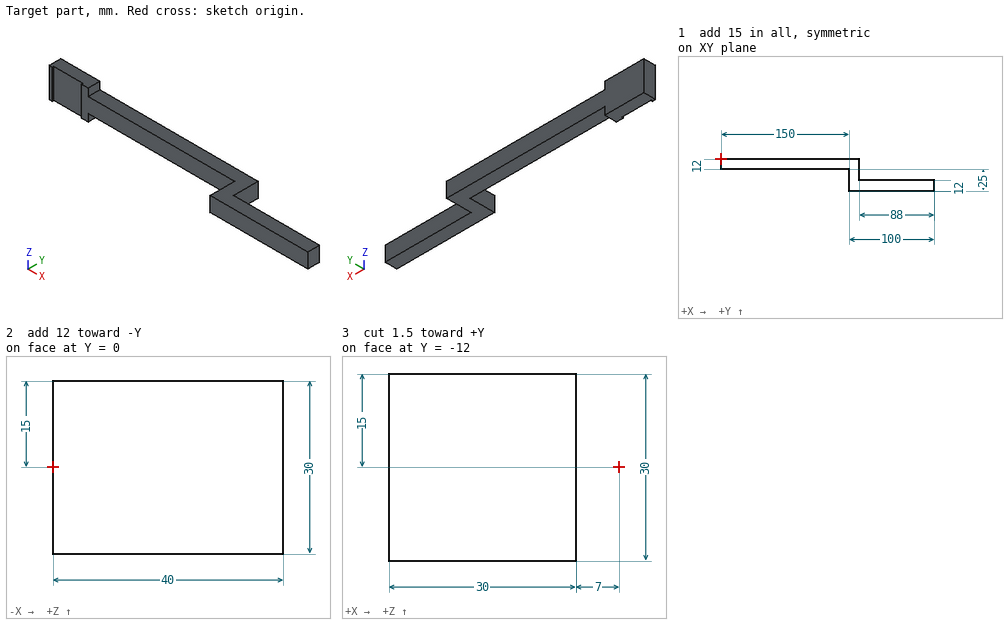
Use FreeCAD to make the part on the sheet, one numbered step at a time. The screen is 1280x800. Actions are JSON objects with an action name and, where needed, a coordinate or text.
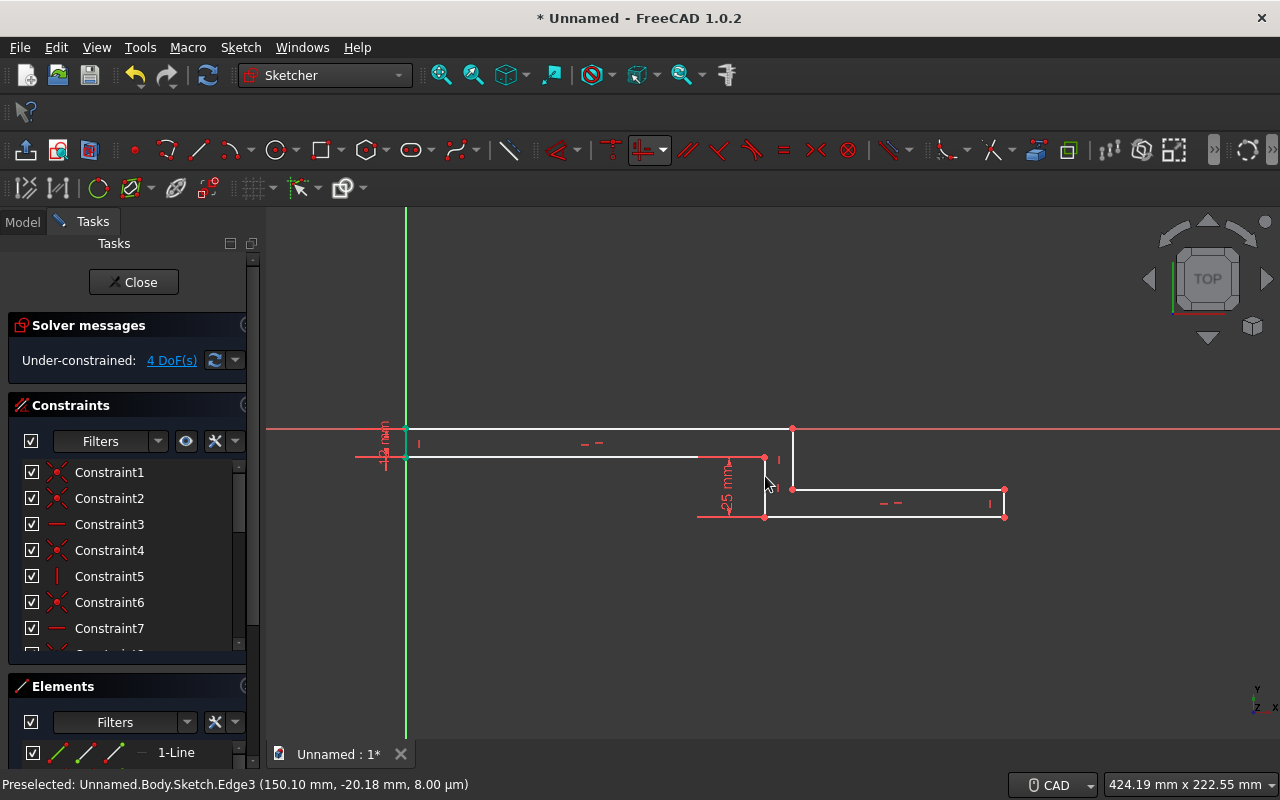
{"action": "scroll", "coordinate": [1004, 506], "scroll_direction": "up", "scroll_amount": 2}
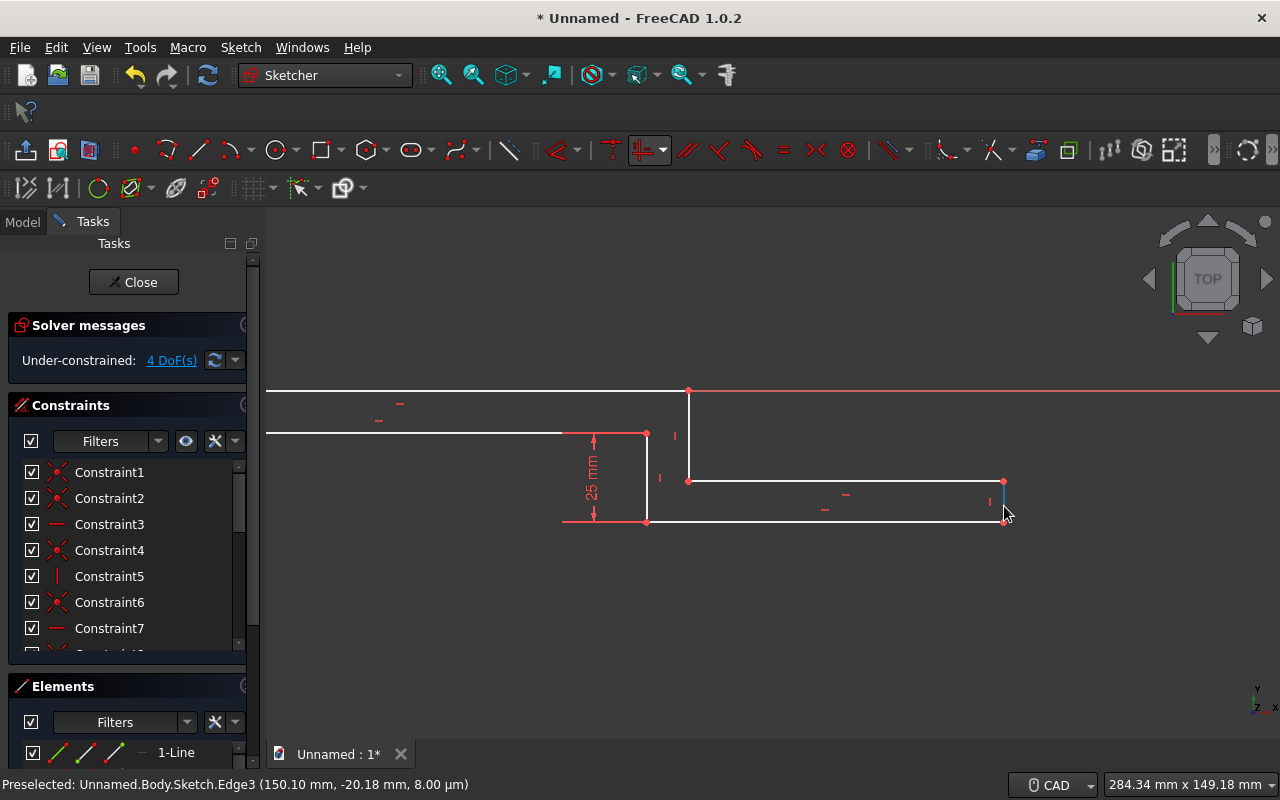
{"action": "left_click", "coordinate": [1004, 506]}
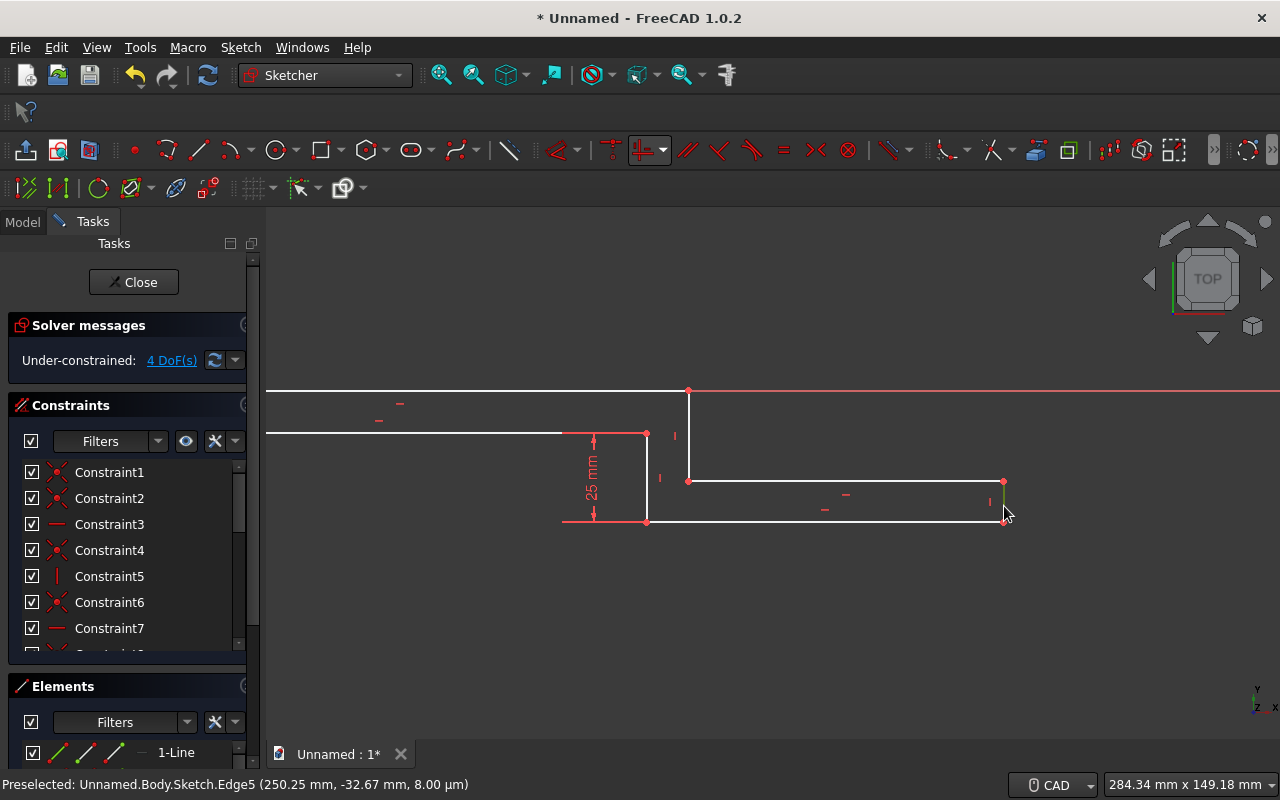
{"action": "left_click", "coordinate": [580, 150]}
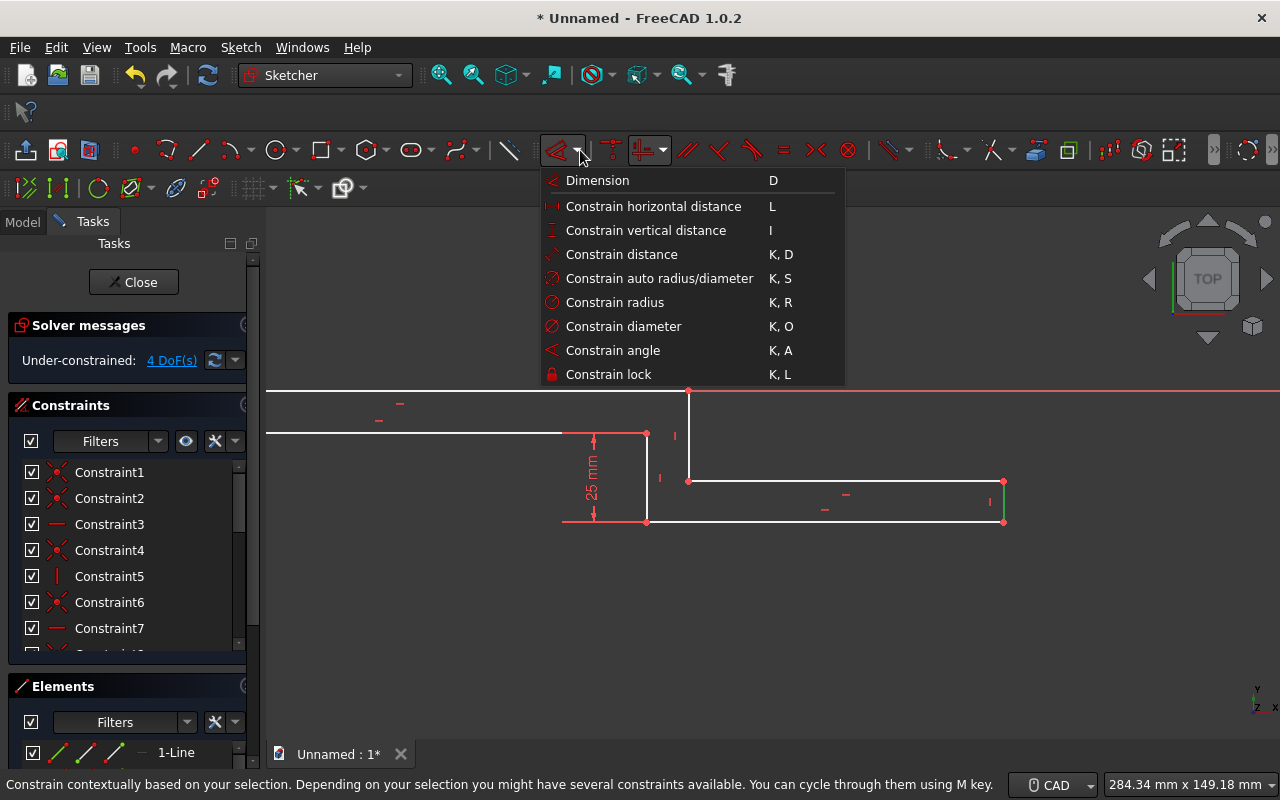
{"action": "left_click", "coordinate": [693, 230]}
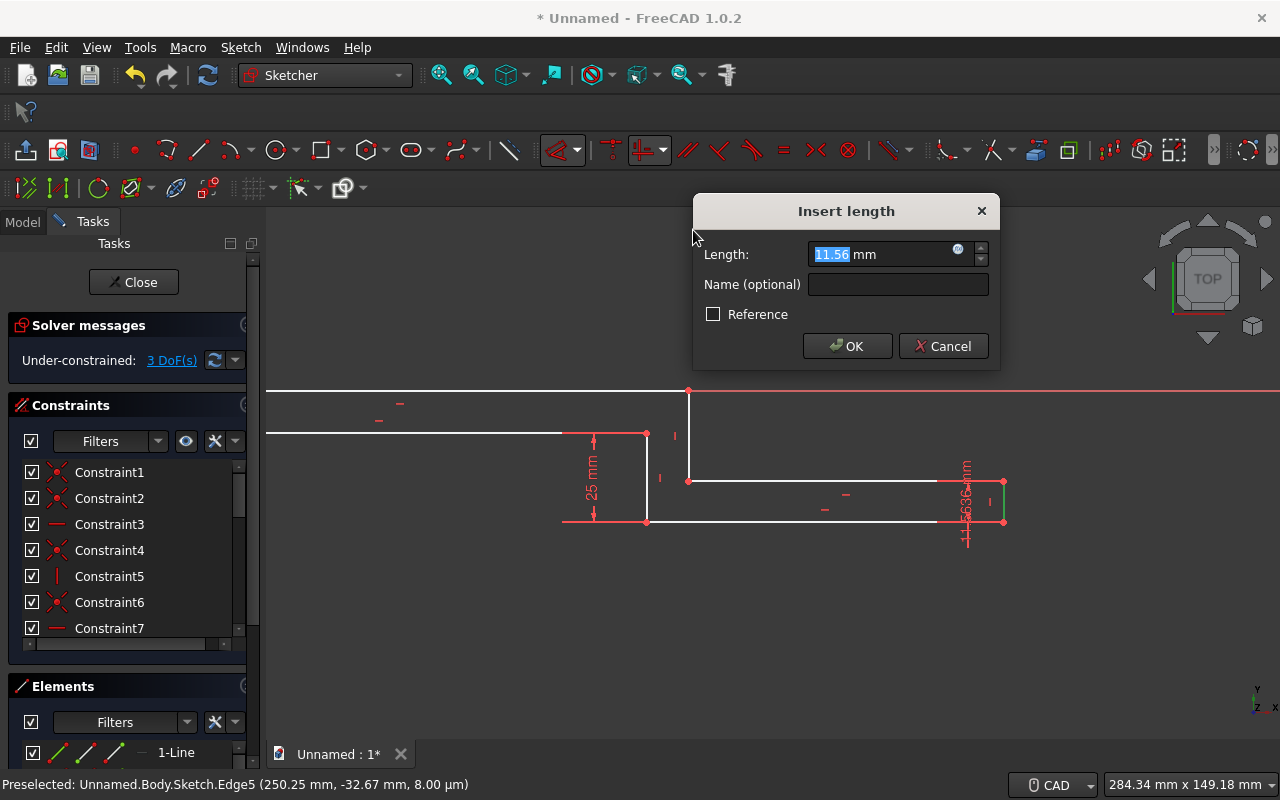
{"action": "type", "text": "12"}
{"action": "key", "text": "Return"}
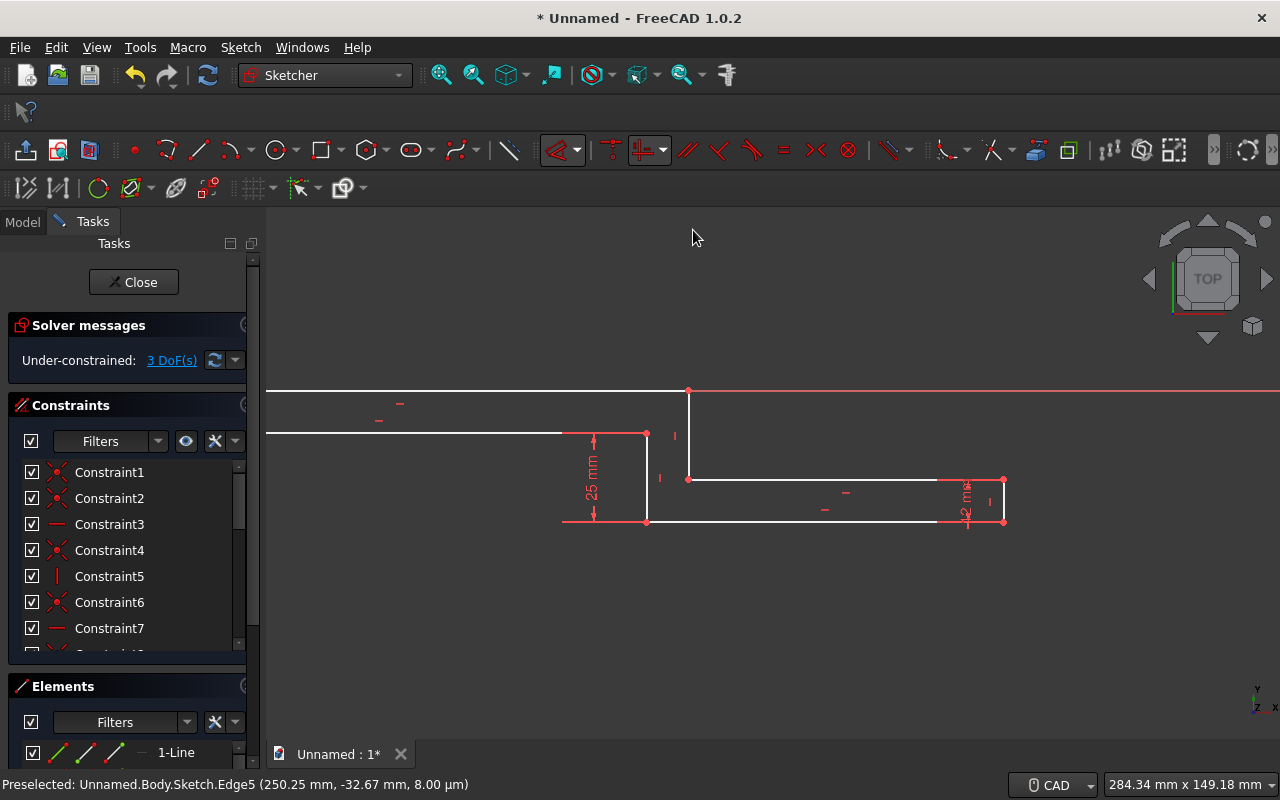
{"action": "left_click", "coordinate": [909, 480]}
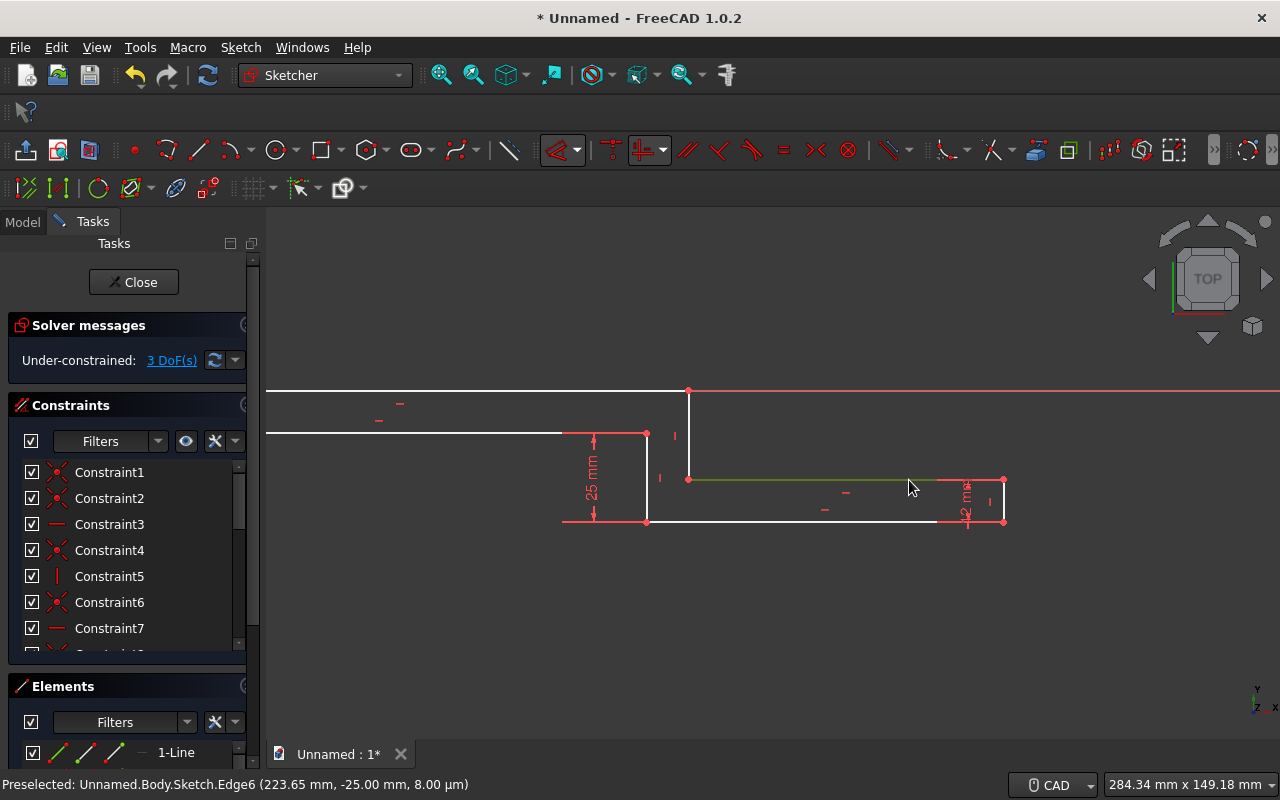
{"action": "key", "text": "l"}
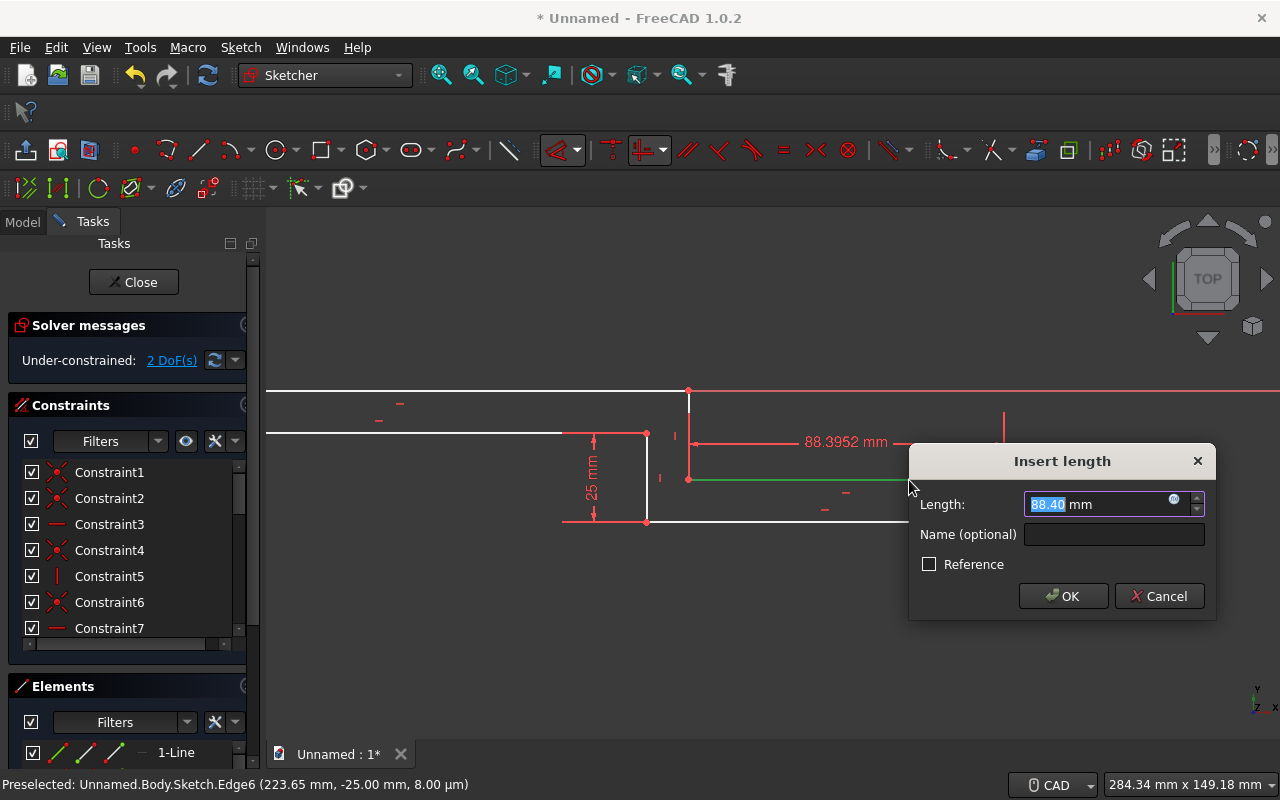
{"action": "type", "text": "88"}
{"action": "key", "text": "Return"}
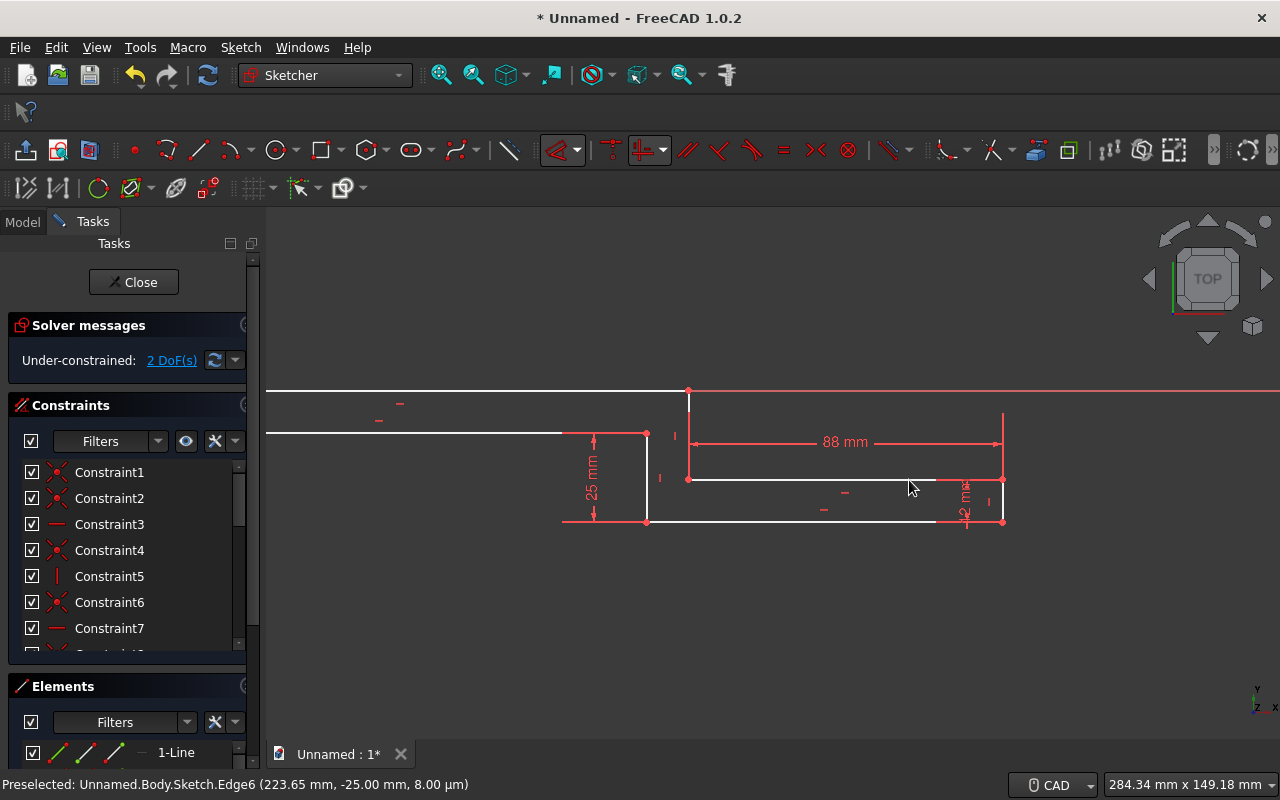
{"action": "left_click", "coordinate": [486, 433]}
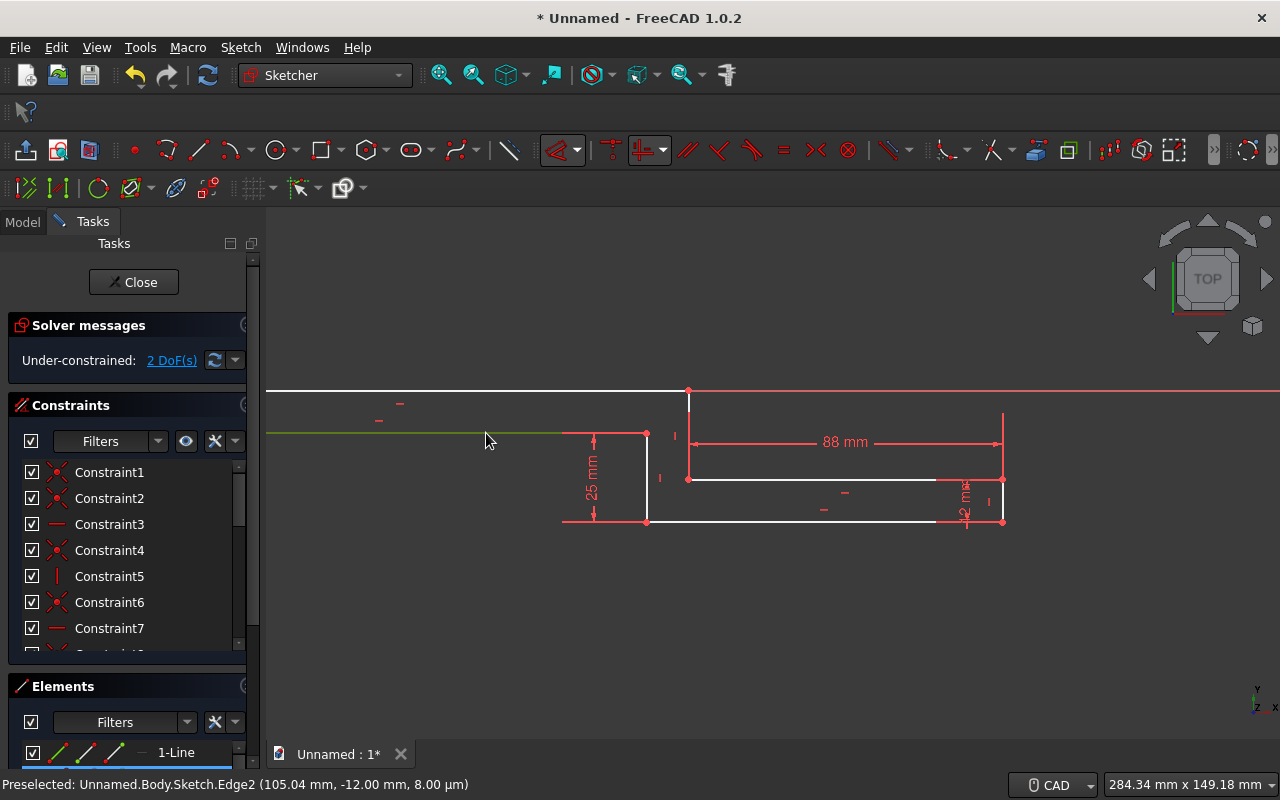
{"action": "left_click", "coordinate": [580, 150]}